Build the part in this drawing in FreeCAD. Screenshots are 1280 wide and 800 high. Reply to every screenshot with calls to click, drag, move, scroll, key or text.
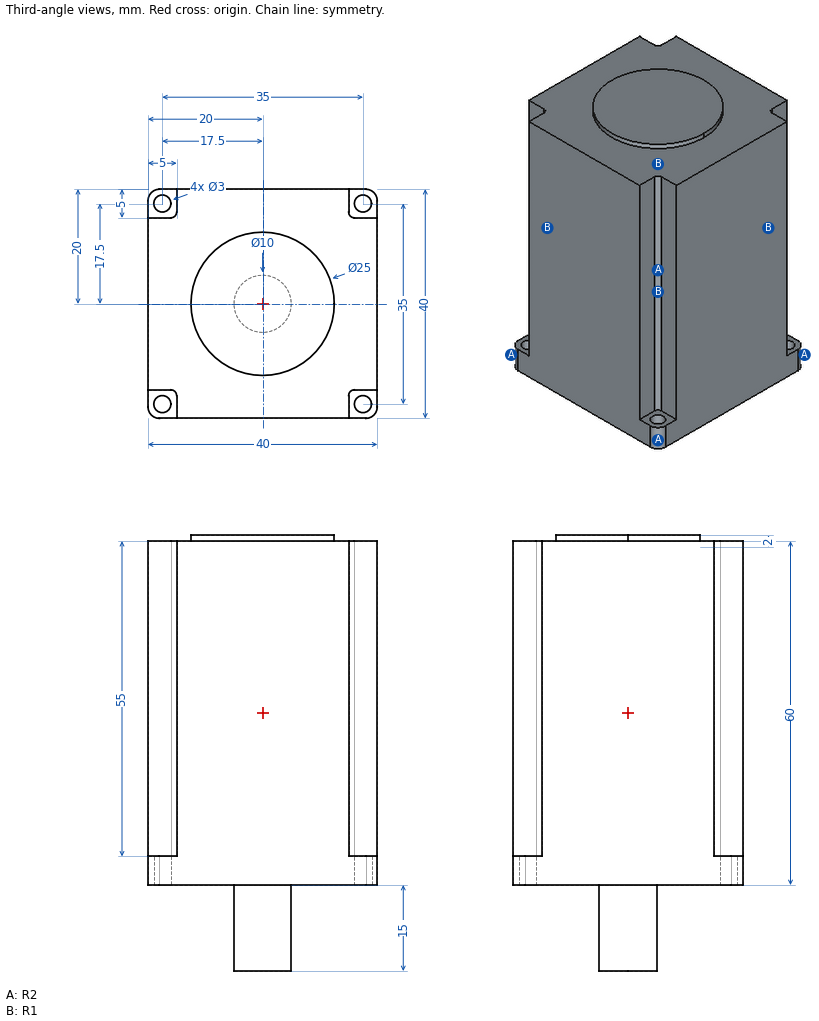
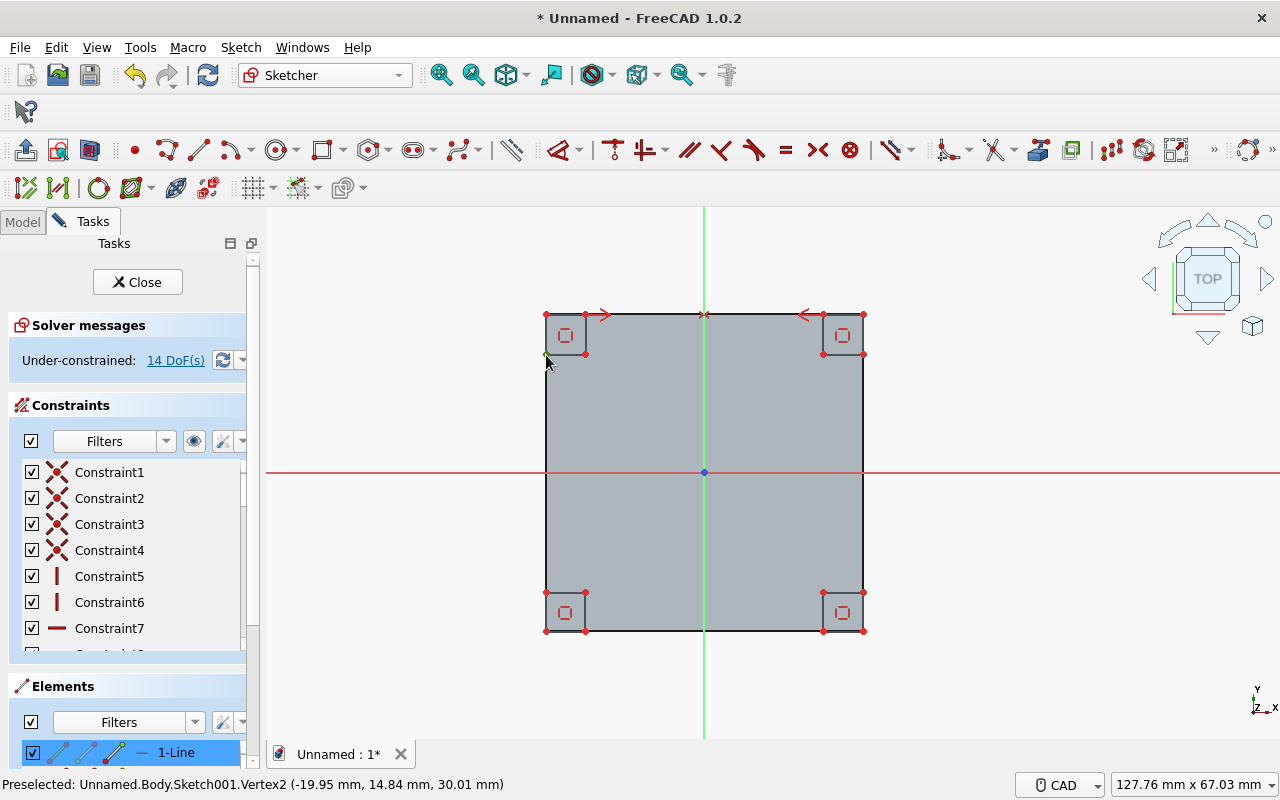
click(863, 355)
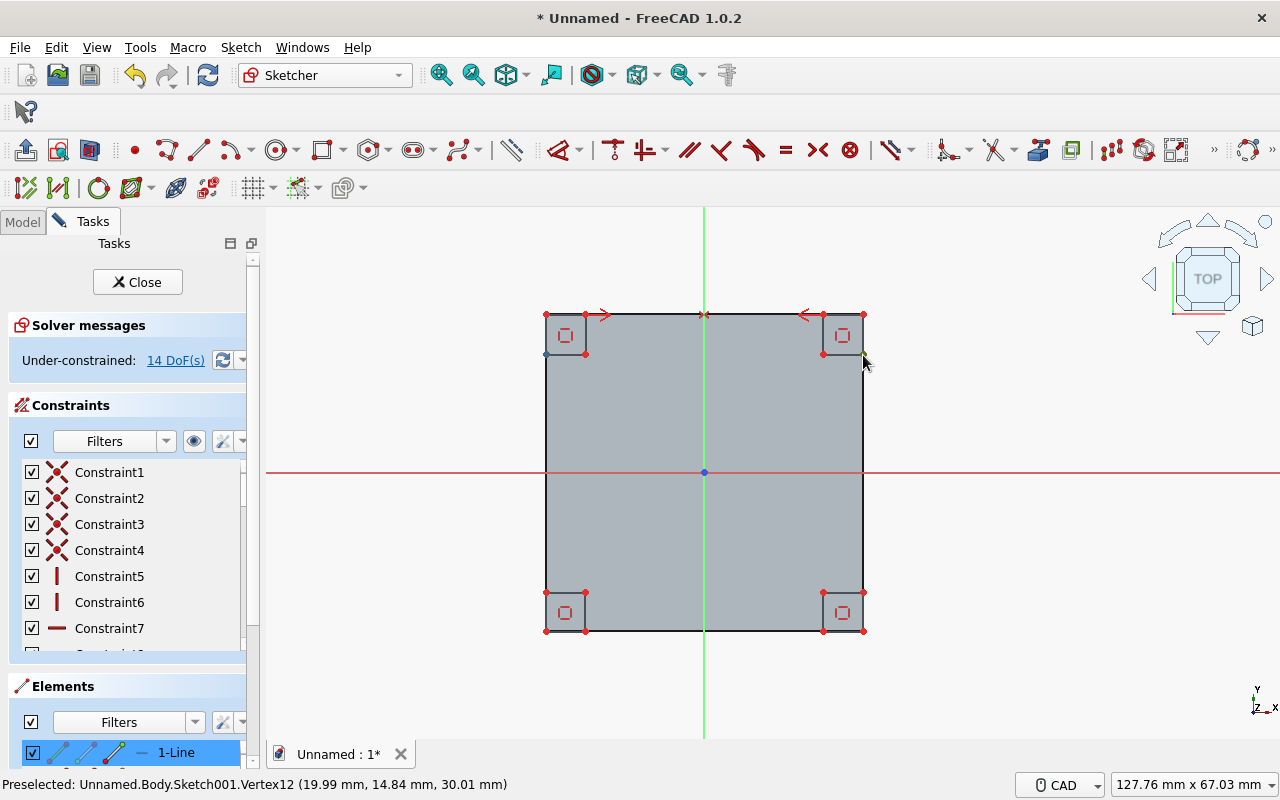
click(704, 677)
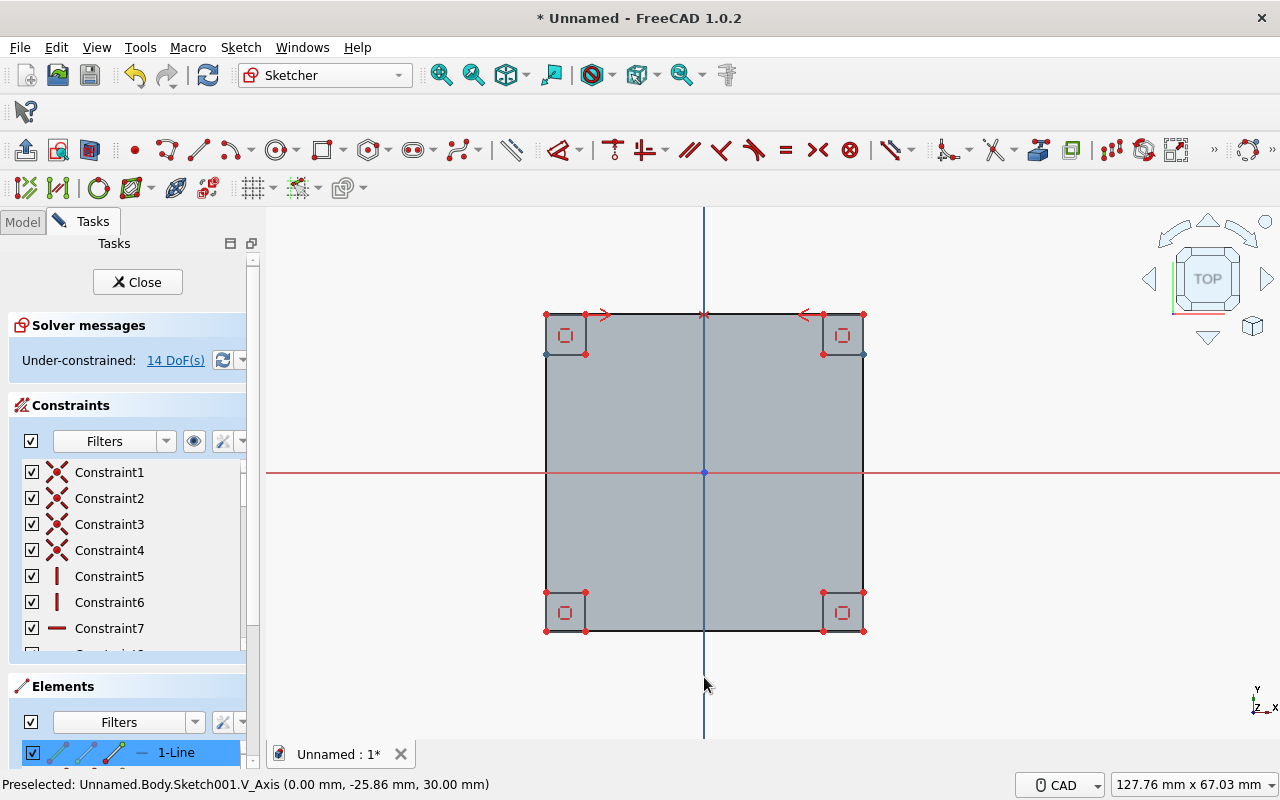
click(818, 150)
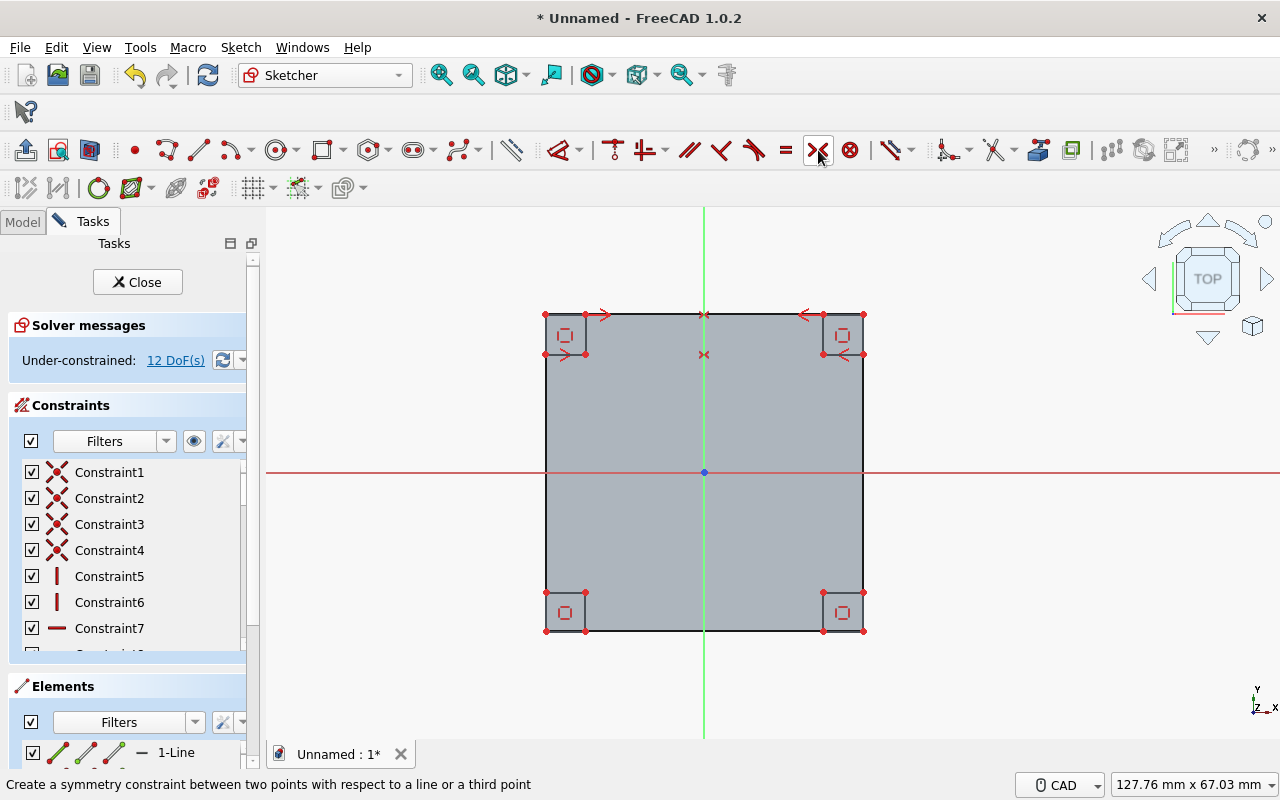
click(823, 355)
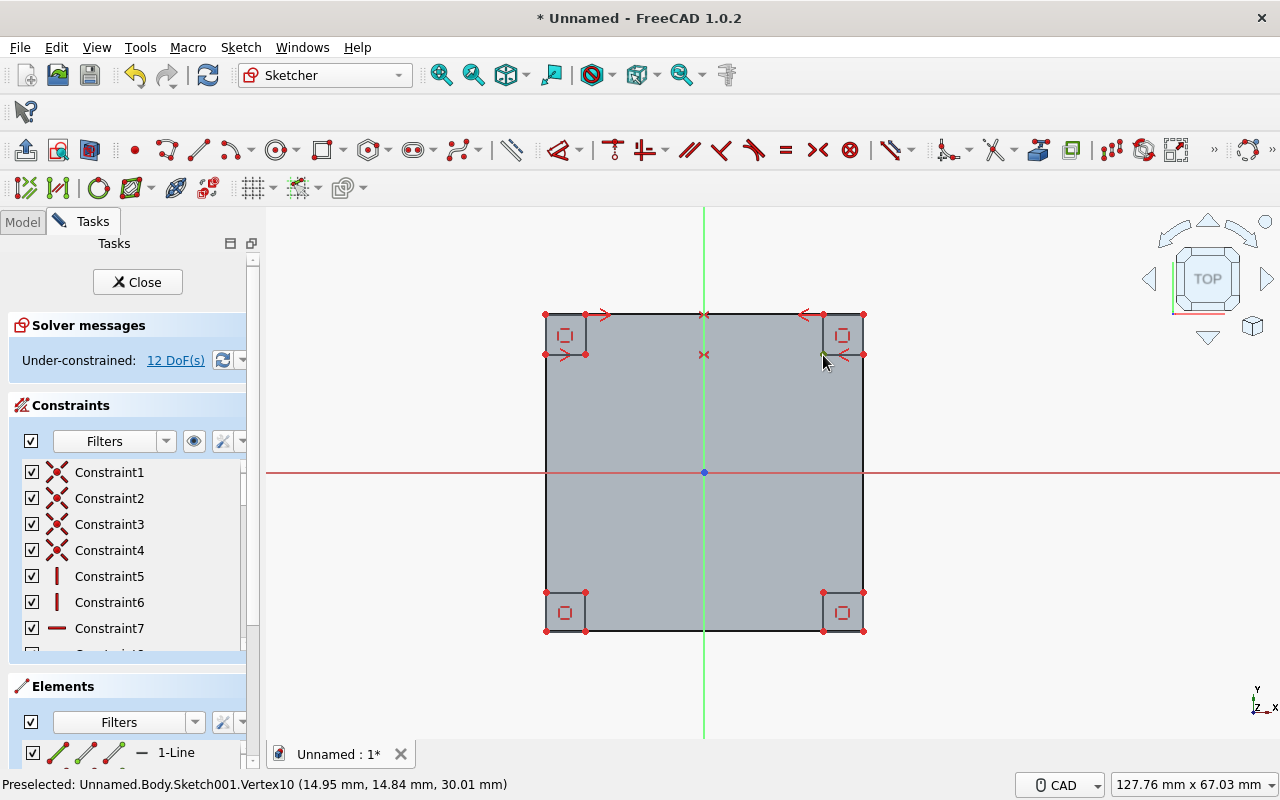
click(823, 593)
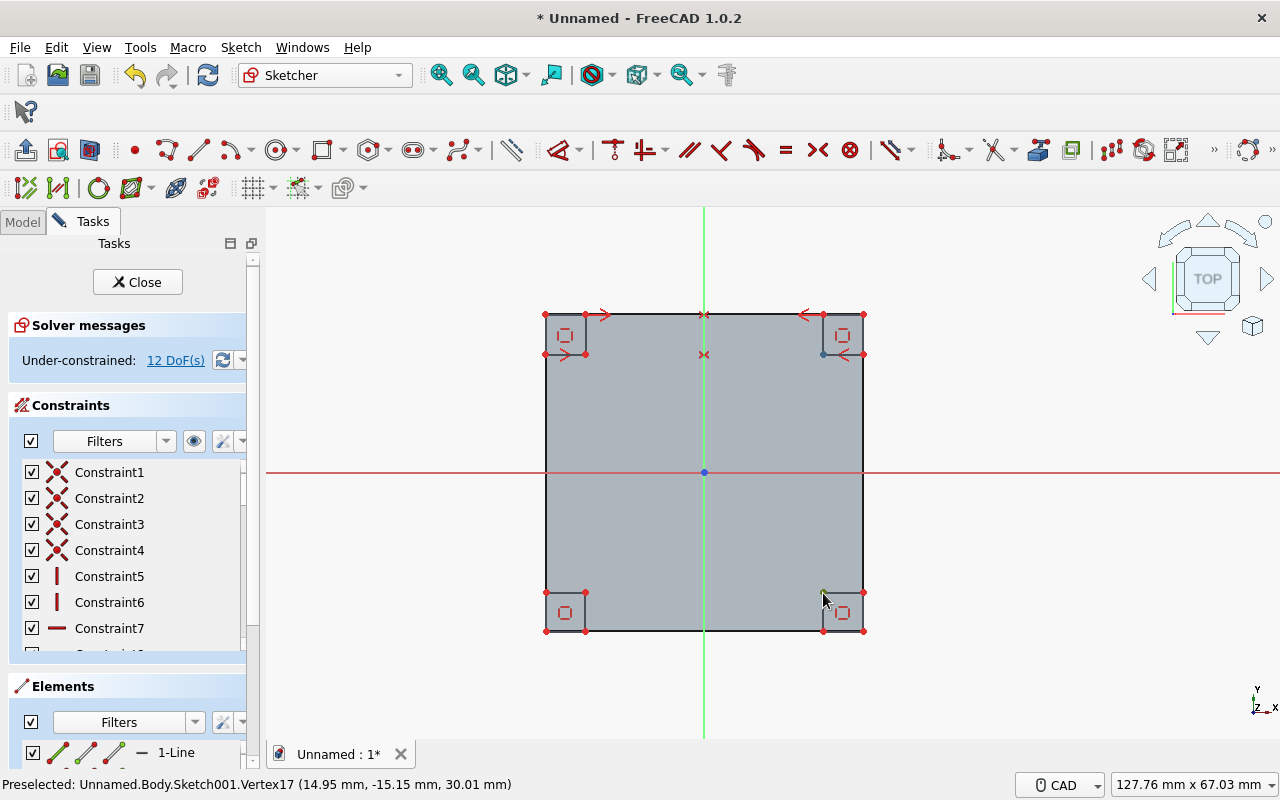
click(353, 473)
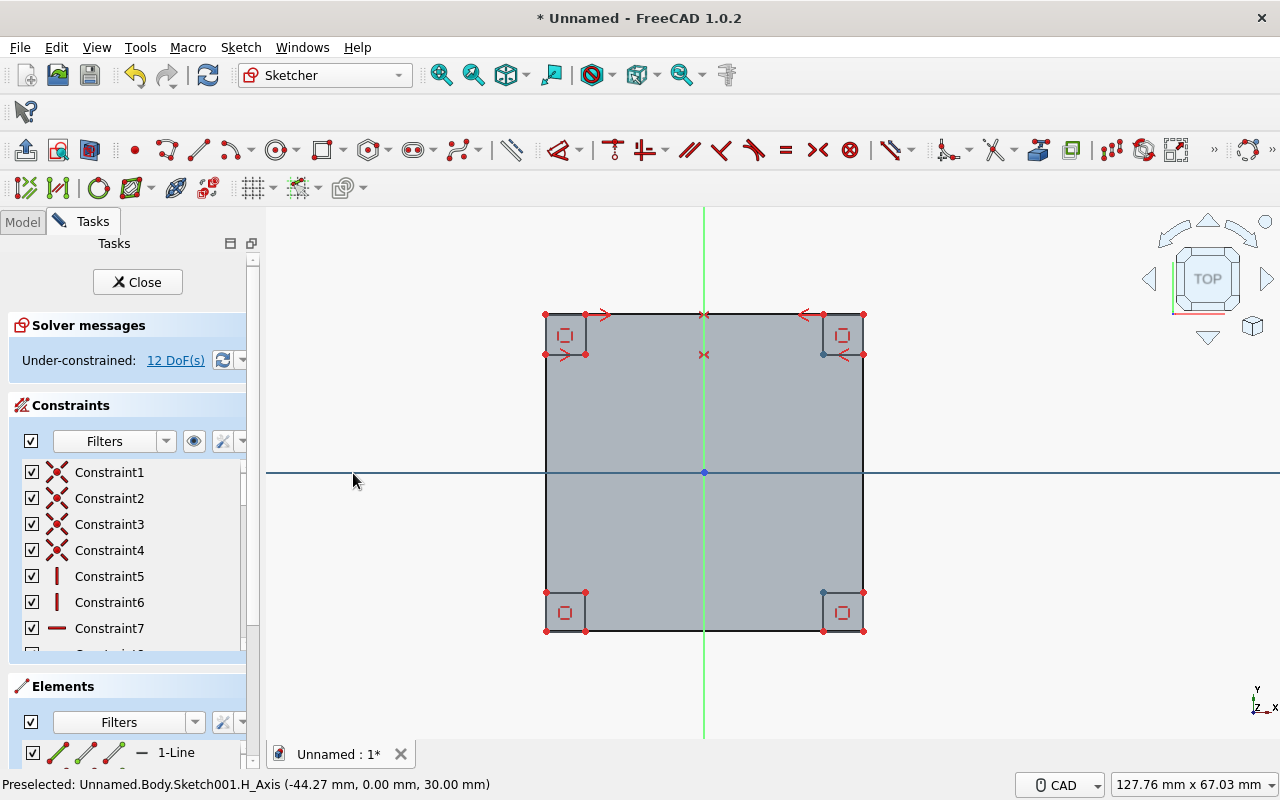
click(818, 150)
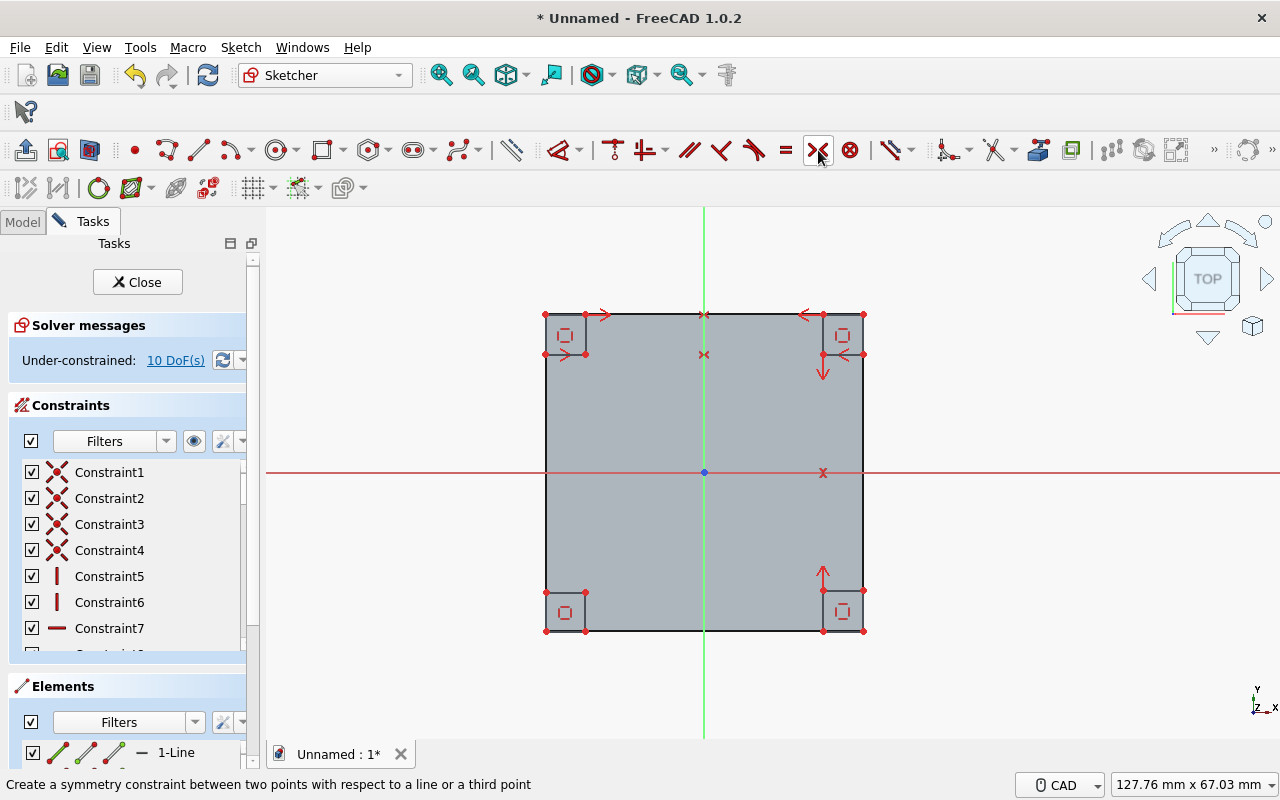
click(863, 315)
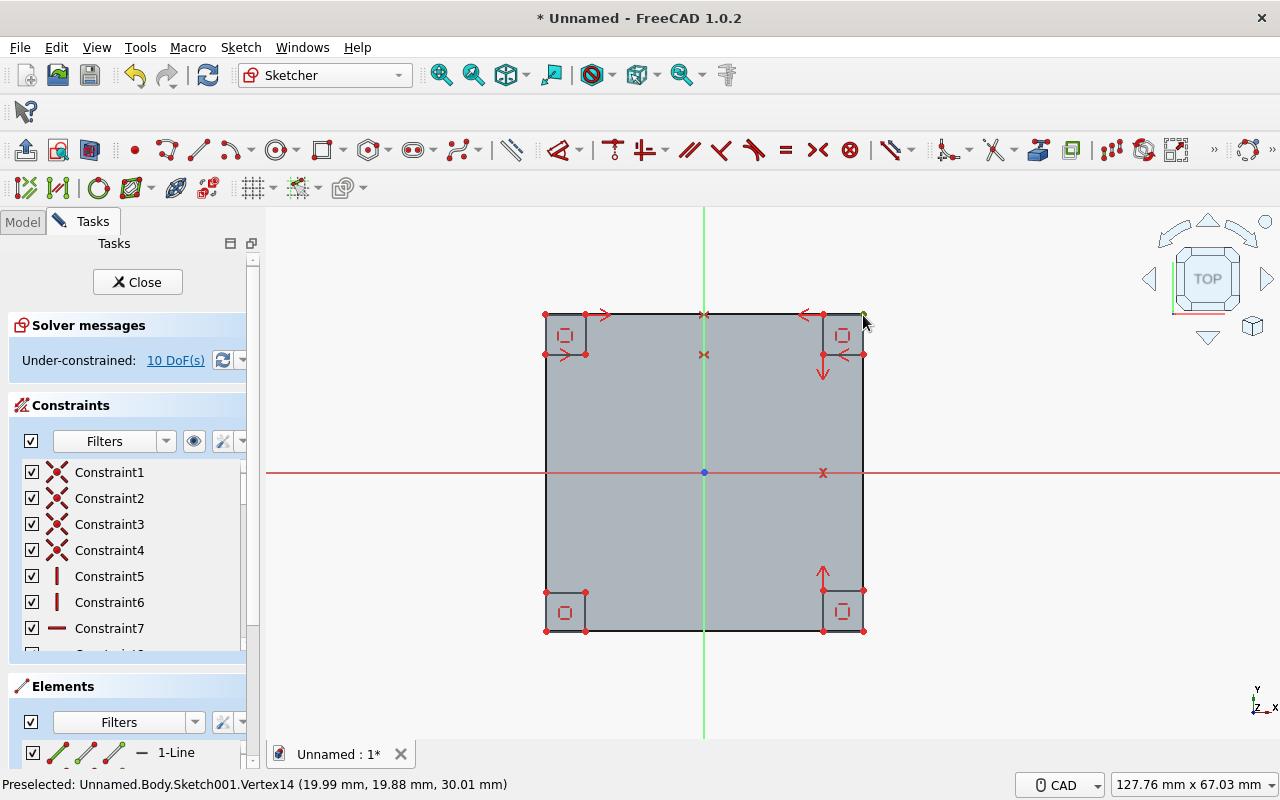
click(863, 632)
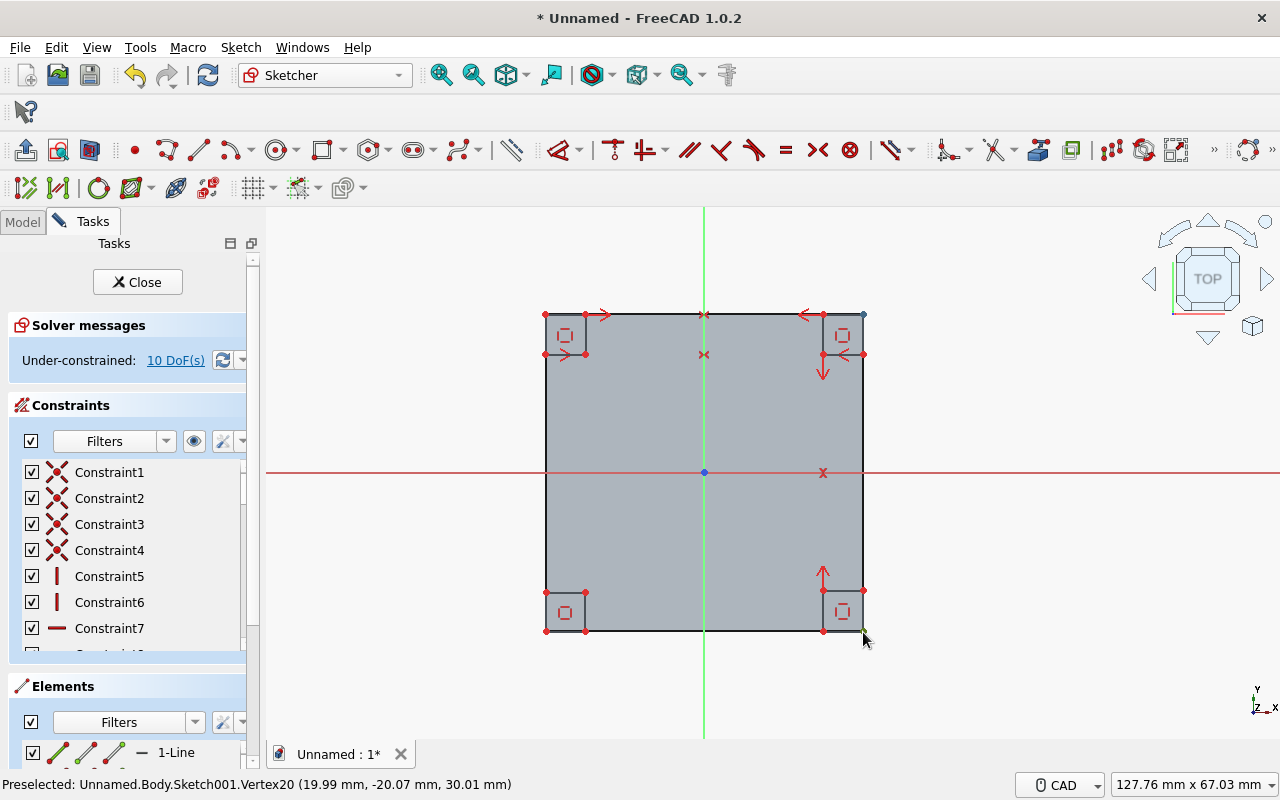
click(353, 473)